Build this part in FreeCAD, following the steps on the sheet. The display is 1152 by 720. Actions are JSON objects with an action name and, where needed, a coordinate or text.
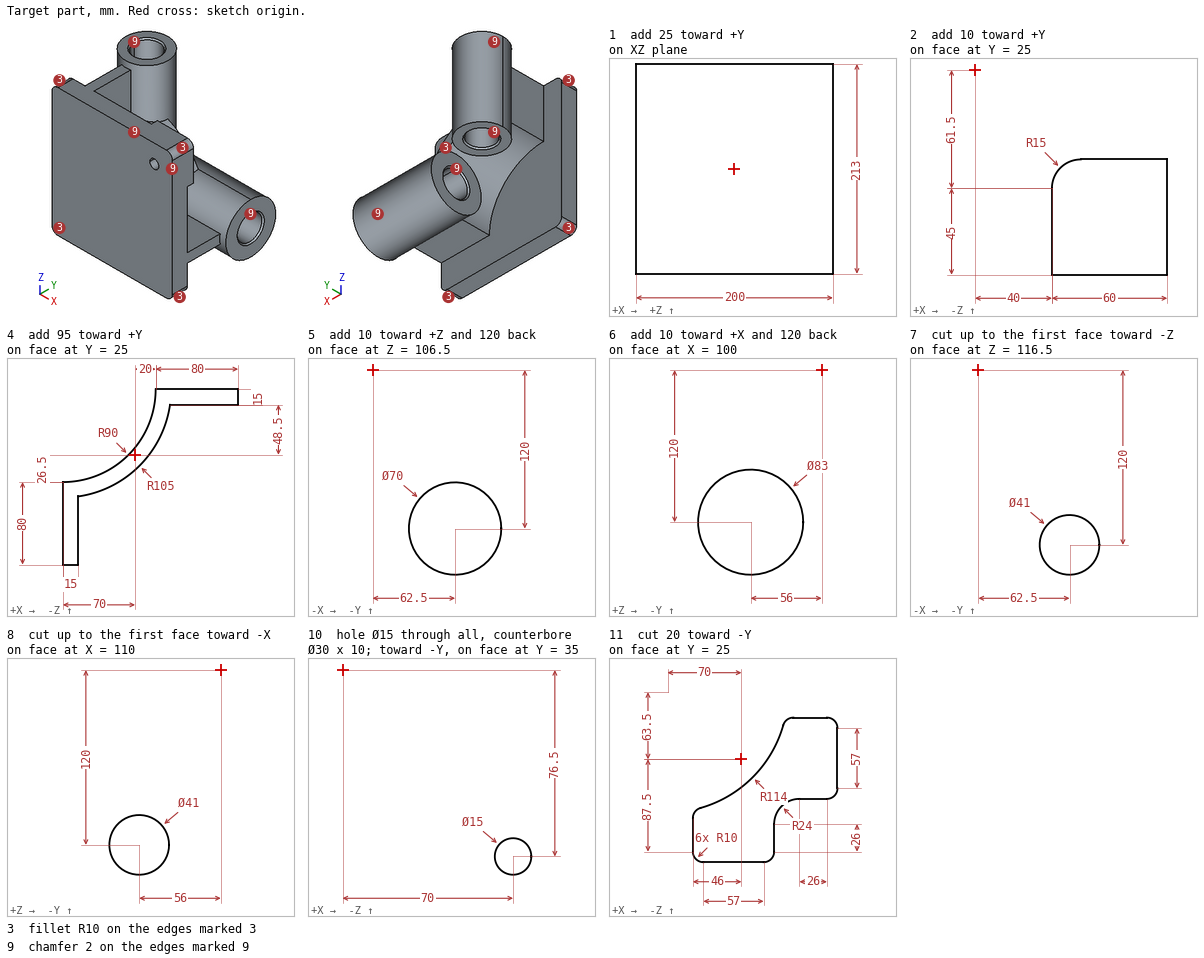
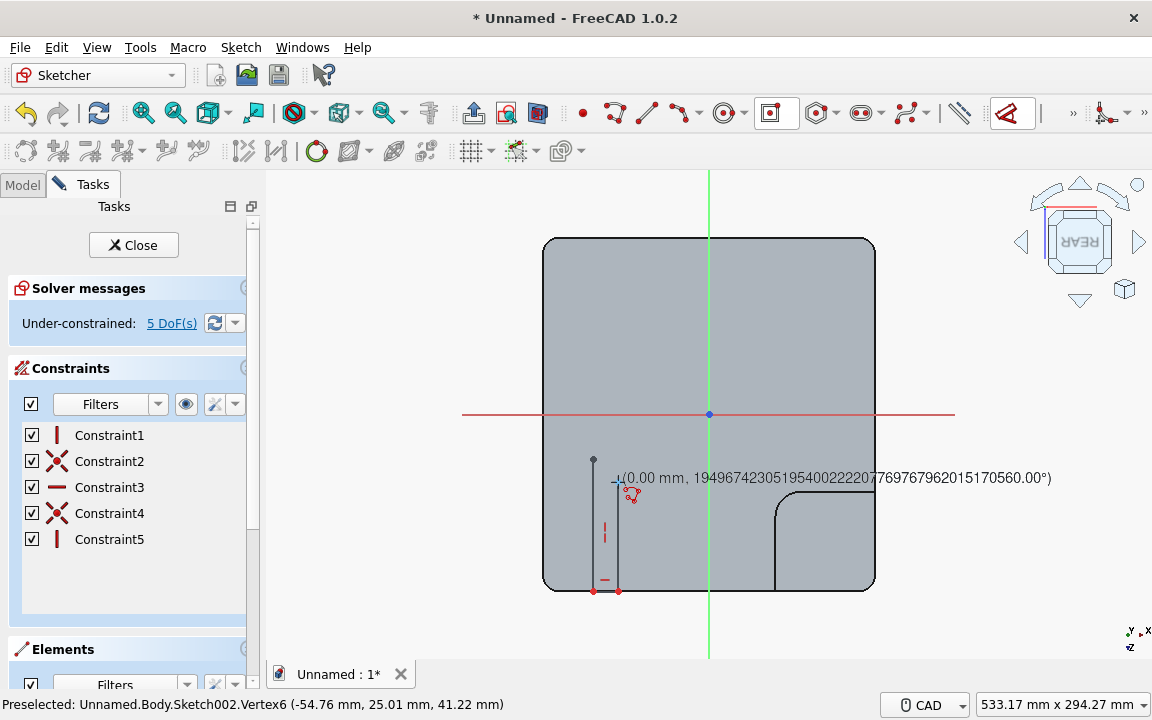
{"action": "left_click", "coordinate": [765, 334]}
{"action": "left_click", "coordinate": [875, 334]}
{"action": "left_click", "coordinate": [875, 309]}
{"action": "left_click", "coordinate": [742, 309]}
{"action": "right_click", "coordinate": [742, 309]}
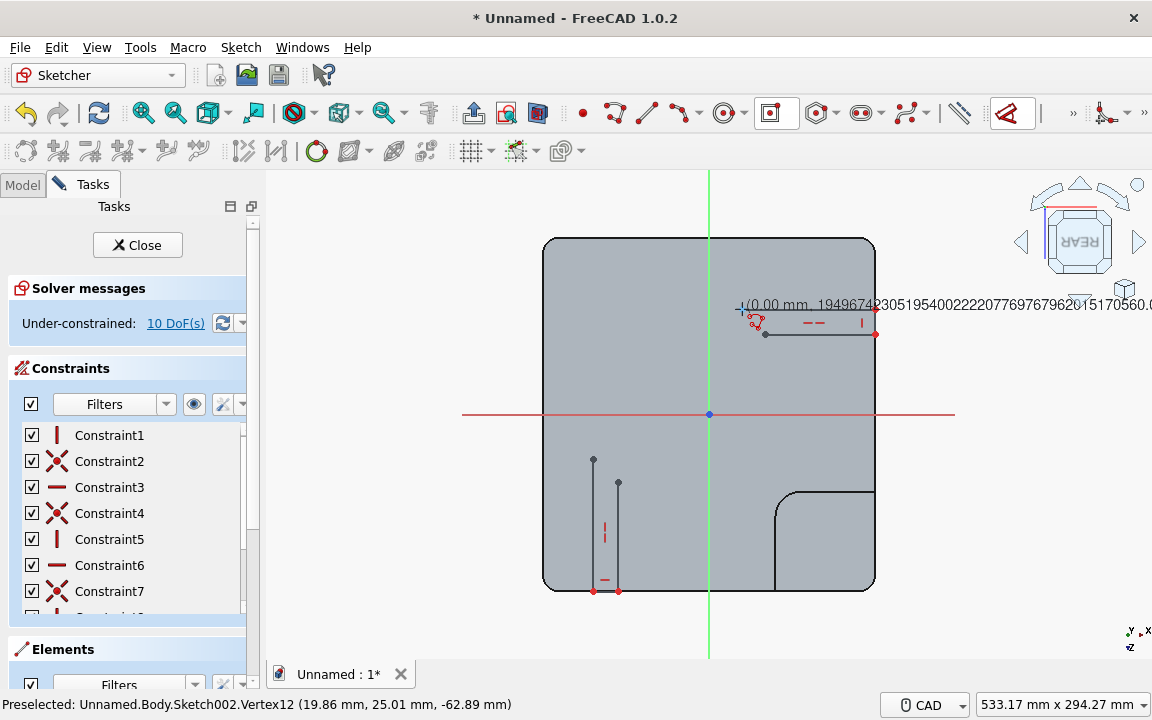
{"action": "left_click", "coordinate": [680, 114]}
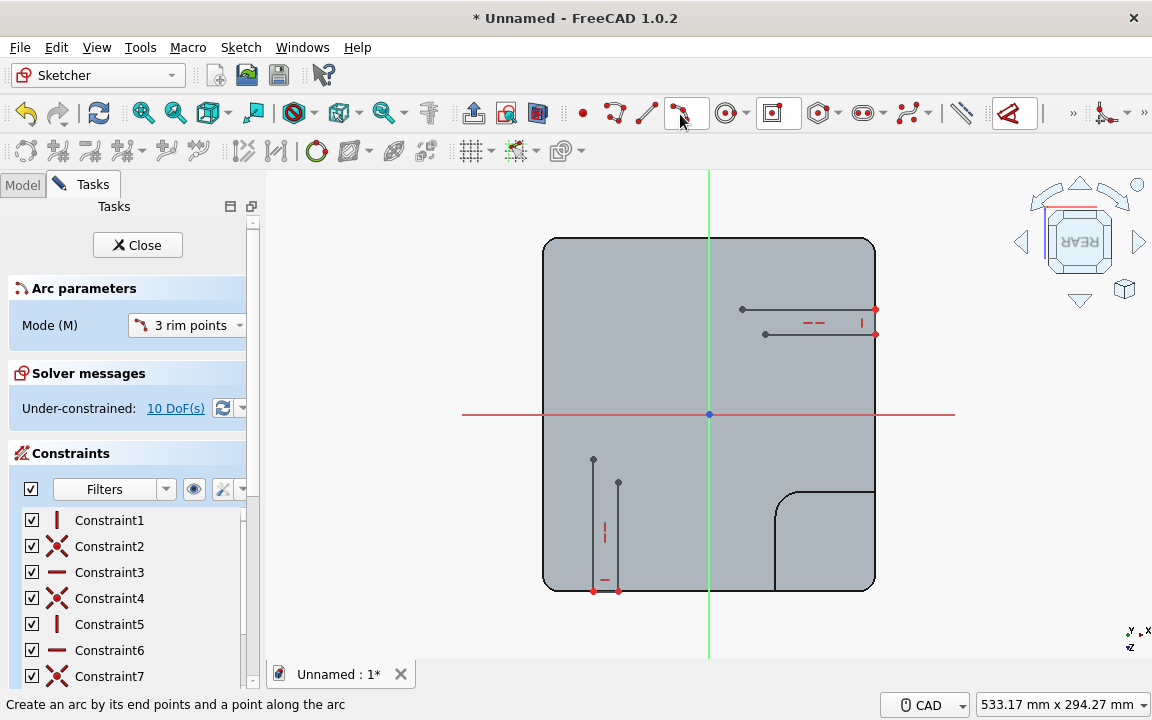
{"action": "left_click", "coordinate": [618, 483]}
{"action": "left_click", "coordinate": [765, 335]}
{"action": "left_click", "coordinate": [681, 460]}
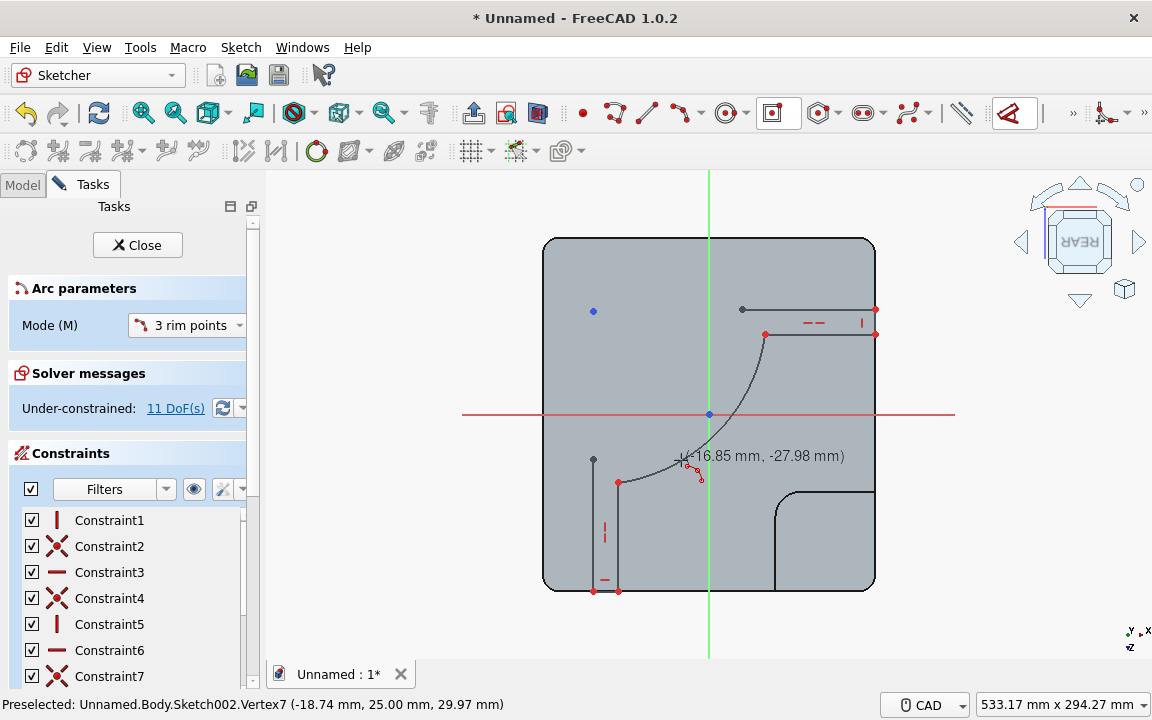
{"action": "left_click", "coordinate": [742, 310]}
{"action": "left_click", "coordinate": [593, 460]}
{"action": "left_click", "coordinate": [681, 430]}
{"action": "key", "text": "Escape"}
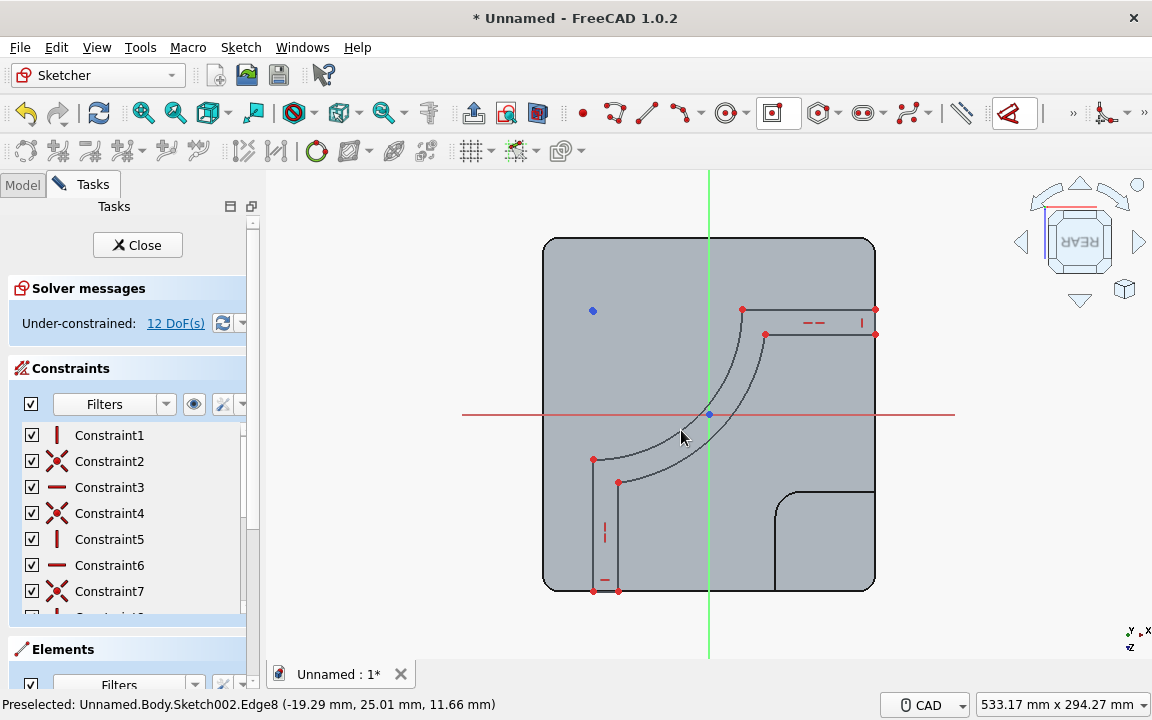
{"action": "left_click", "coordinate": [681, 461]}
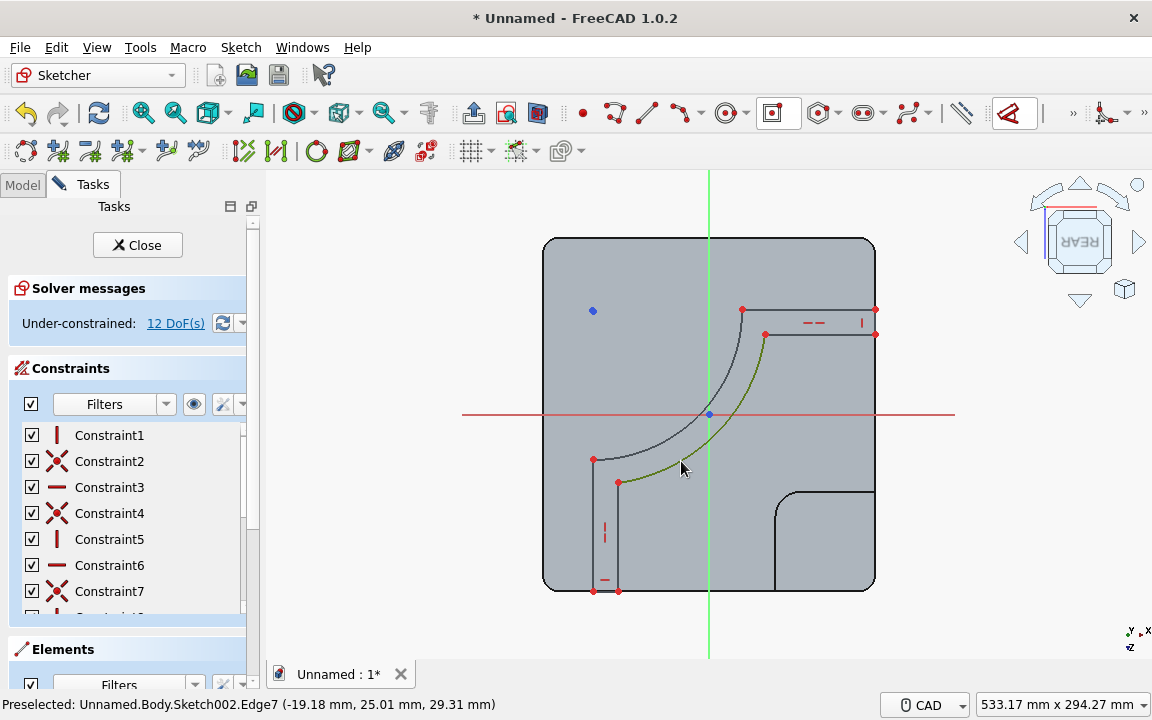
{"action": "left_click", "coordinate": [661, 443]}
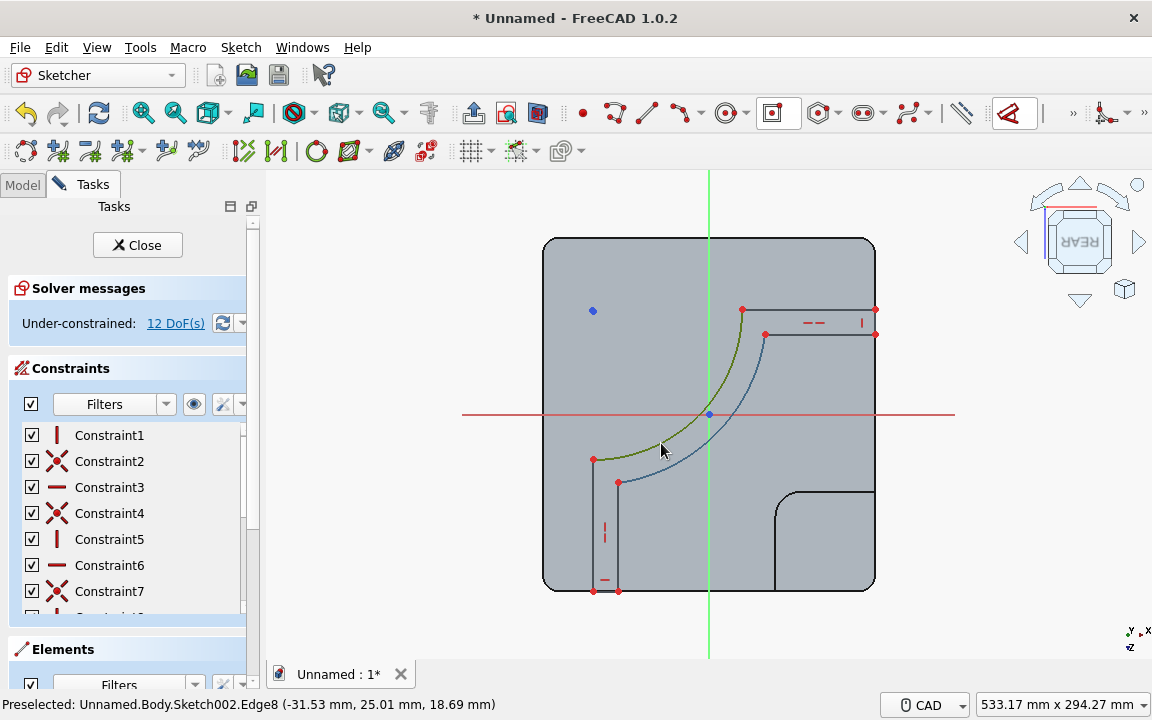
{"action": "key", "text": "c"}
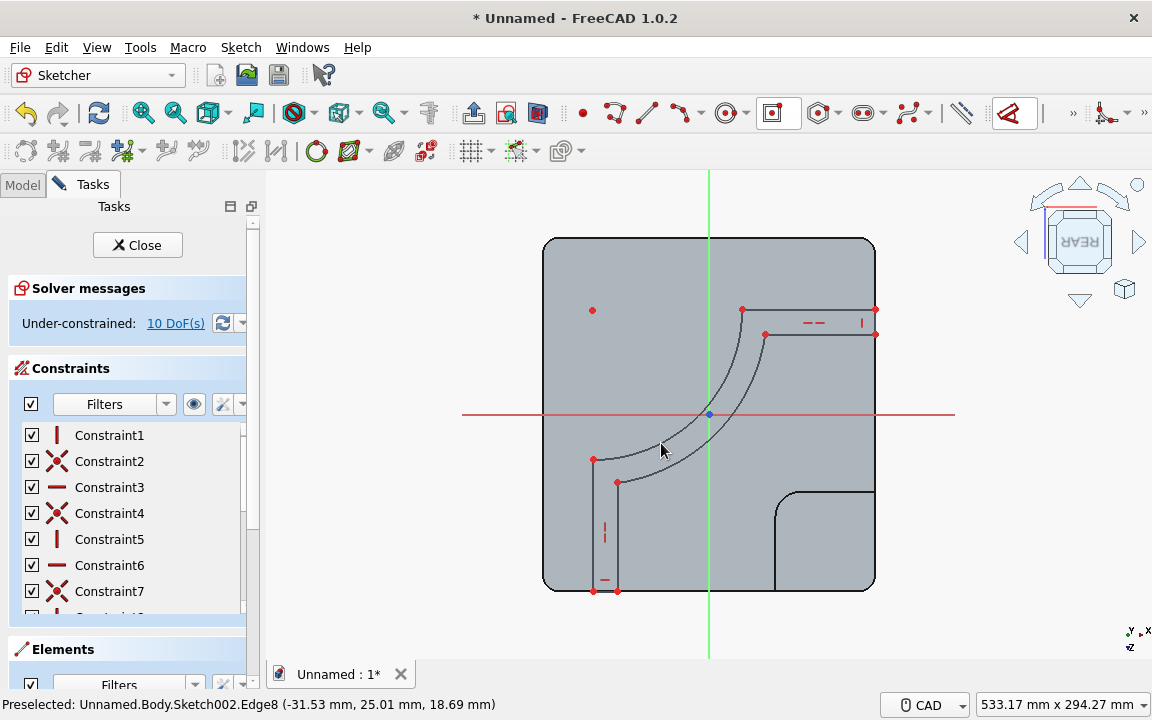
{"action": "left_click", "coordinate": [681, 461]}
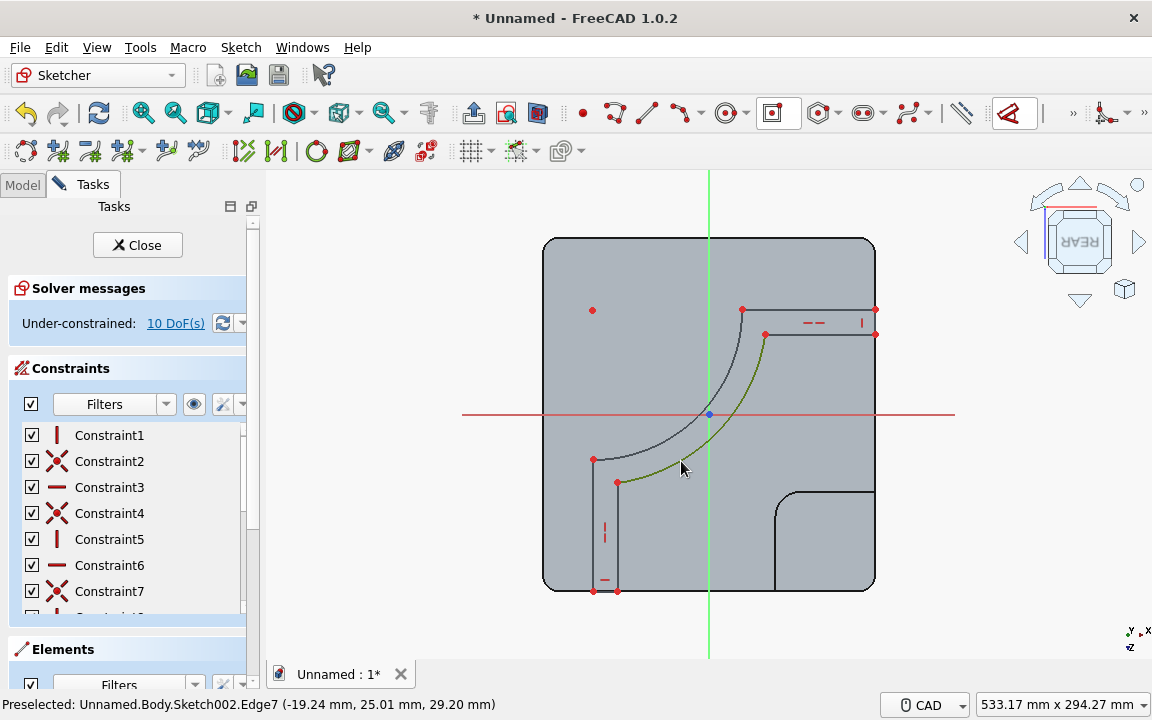
{"action": "key", "text": "k r"}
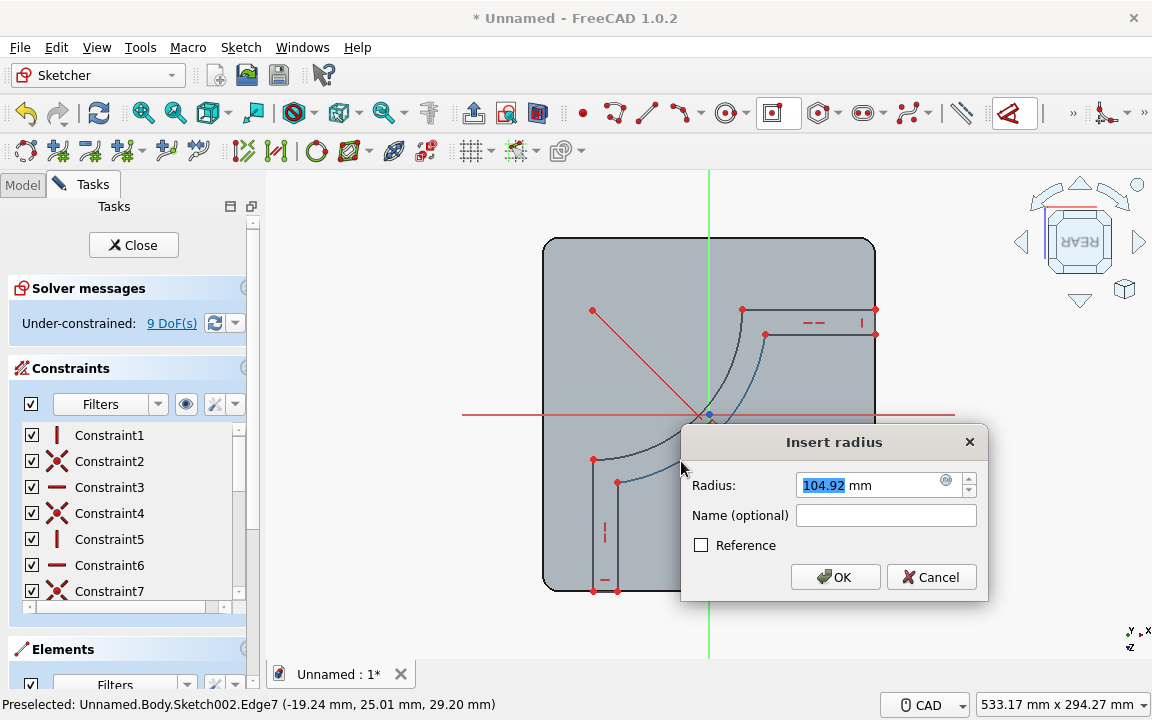
{"action": "type", "text": "105"}
{"action": "key", "text": "Return"}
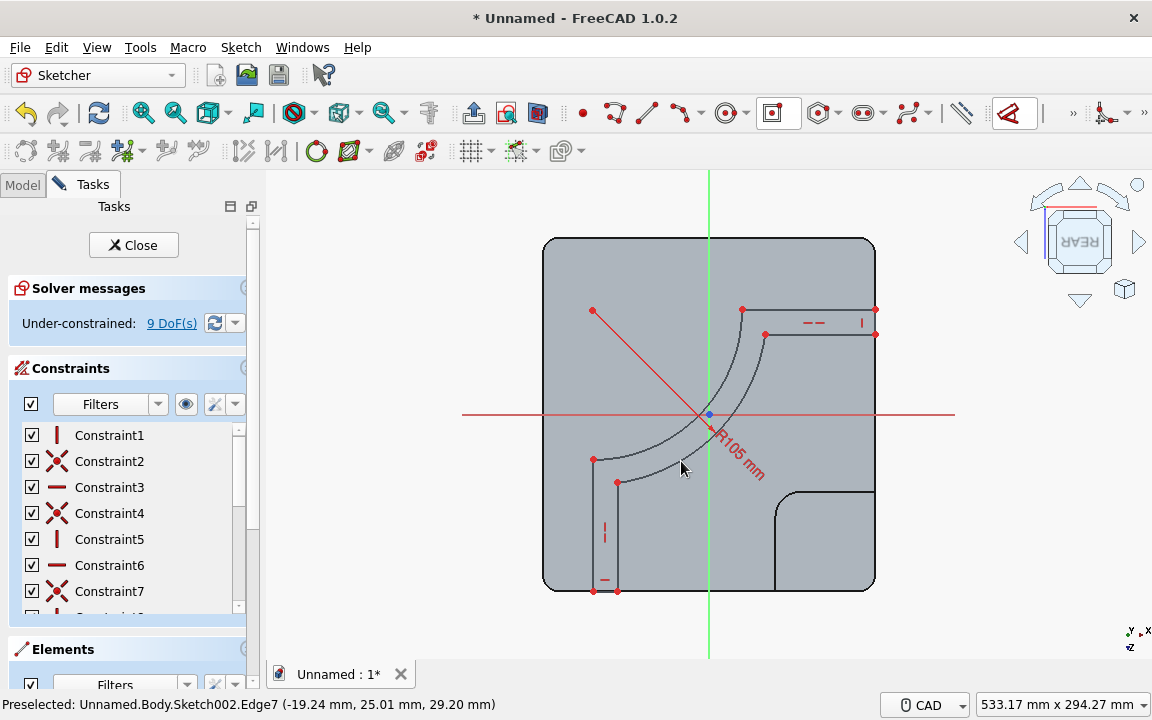
{"action": "left_click", "coordinate": [661, 443]}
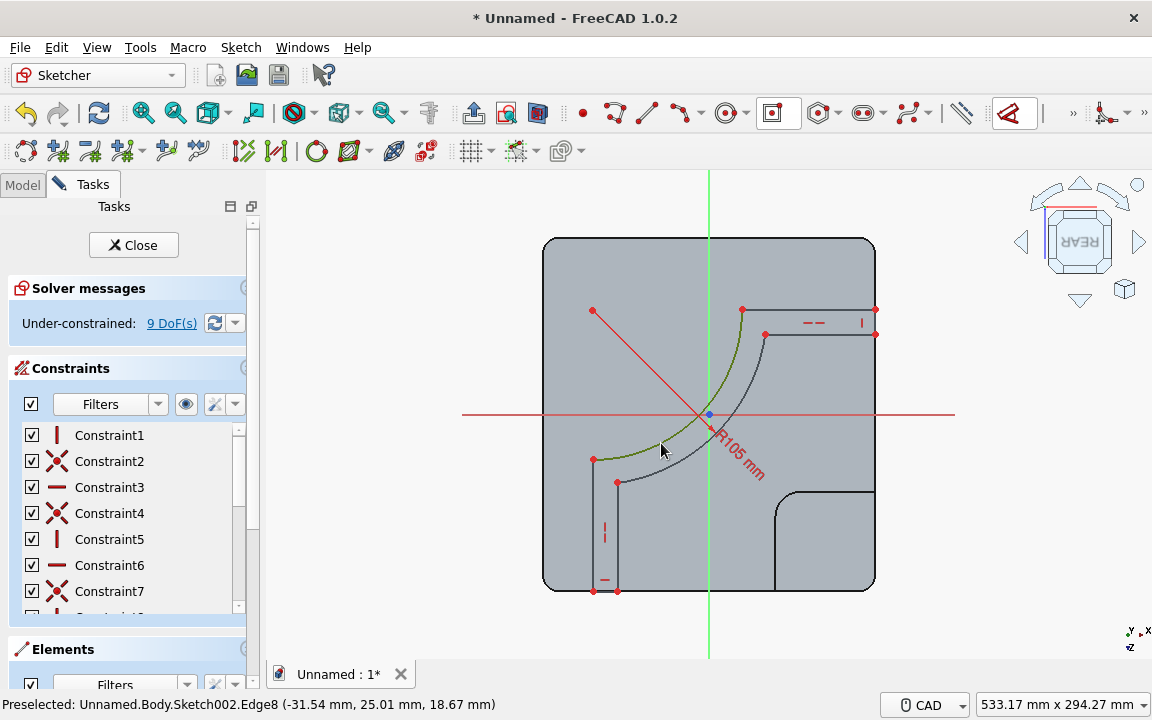
{"action": "key", "text": "k r"}